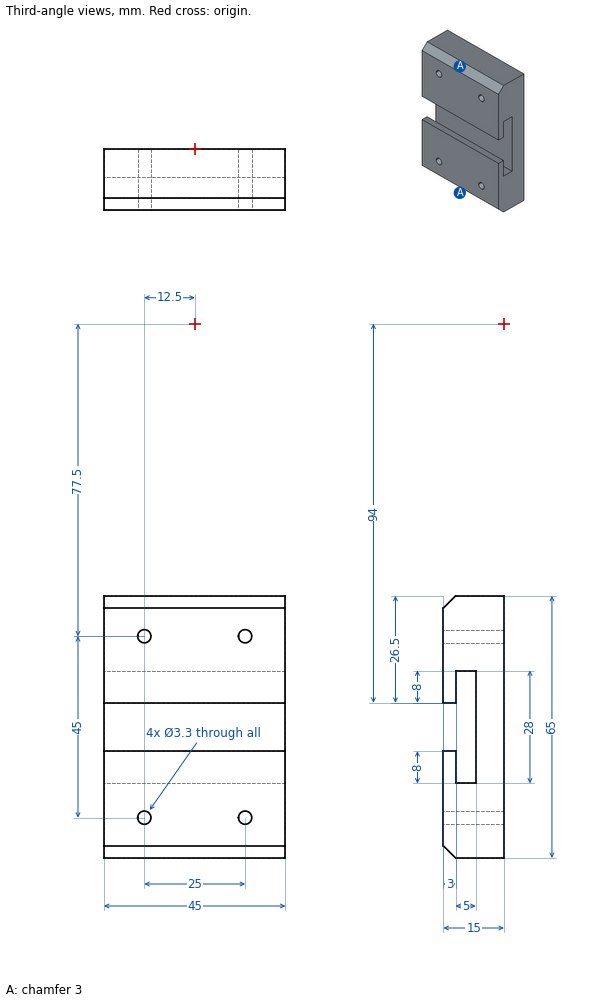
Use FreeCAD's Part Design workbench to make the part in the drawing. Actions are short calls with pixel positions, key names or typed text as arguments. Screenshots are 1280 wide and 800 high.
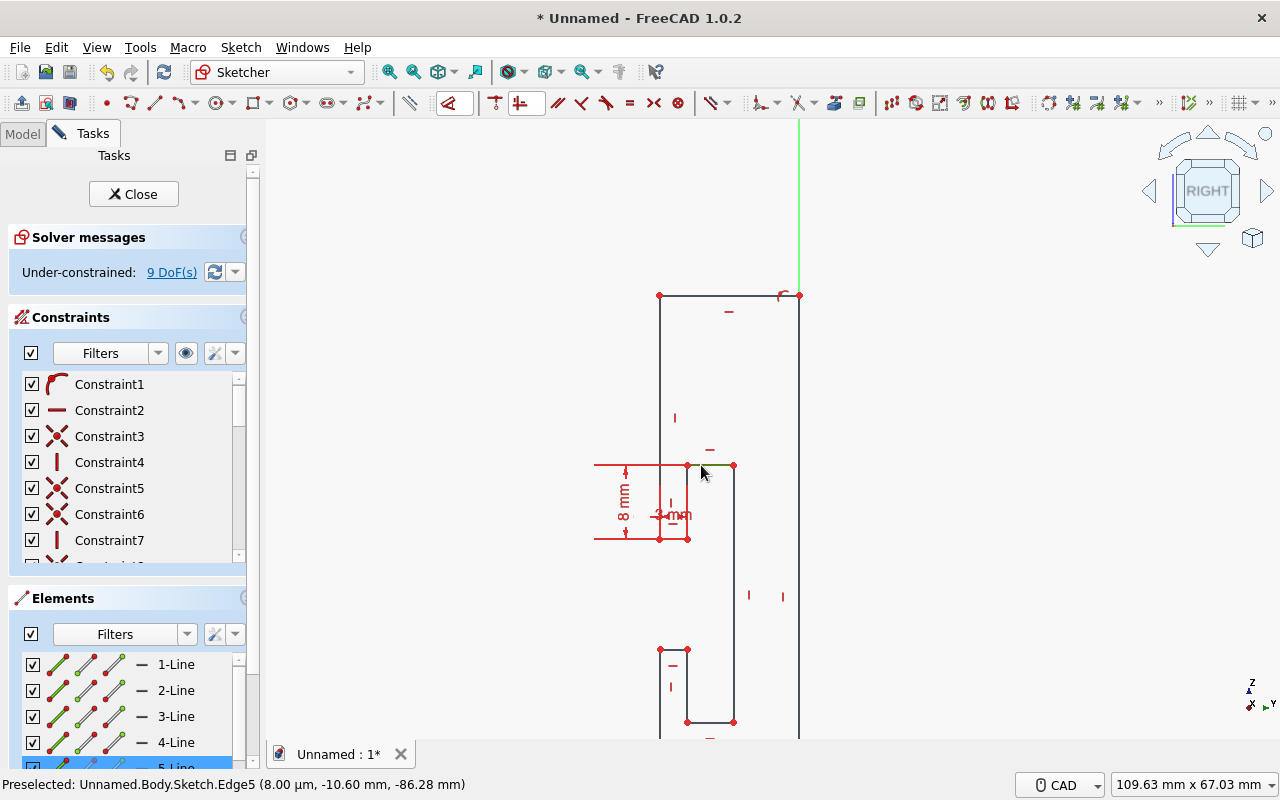
key(l)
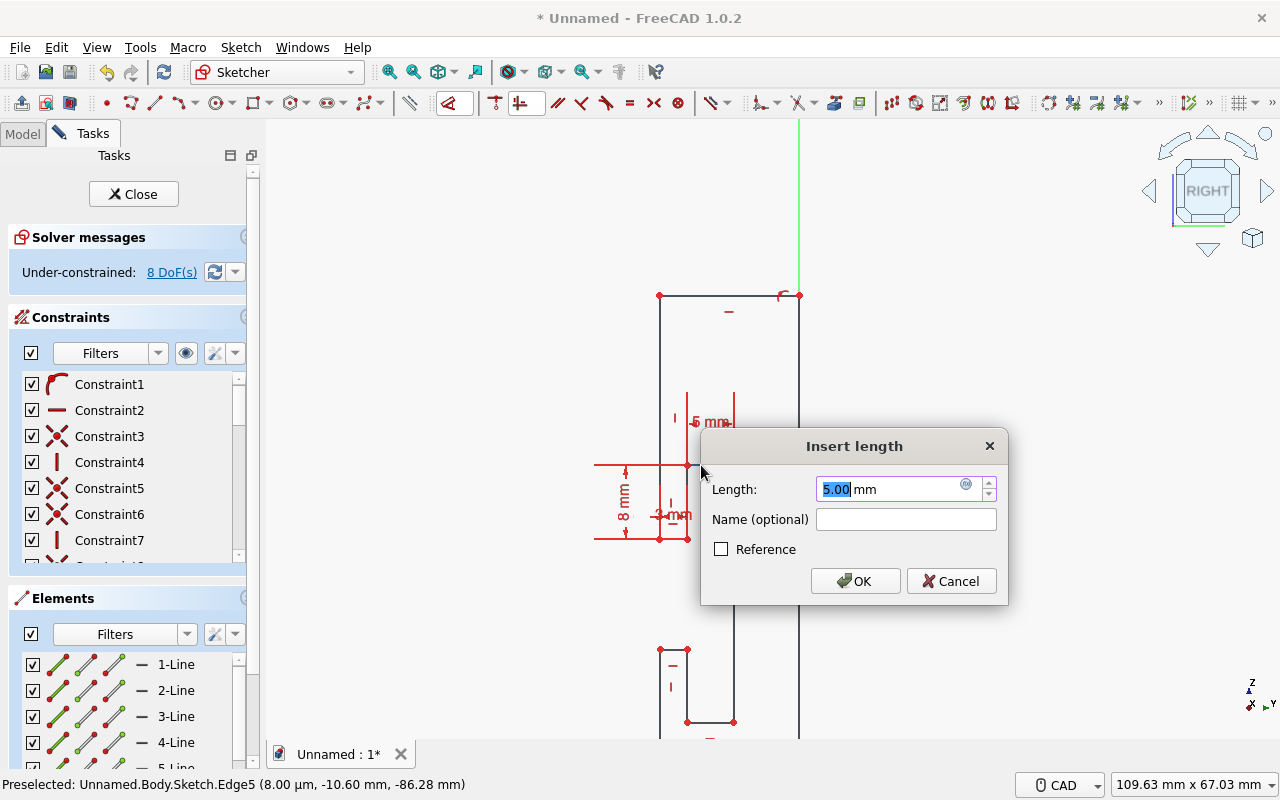
text(5)
key(Return)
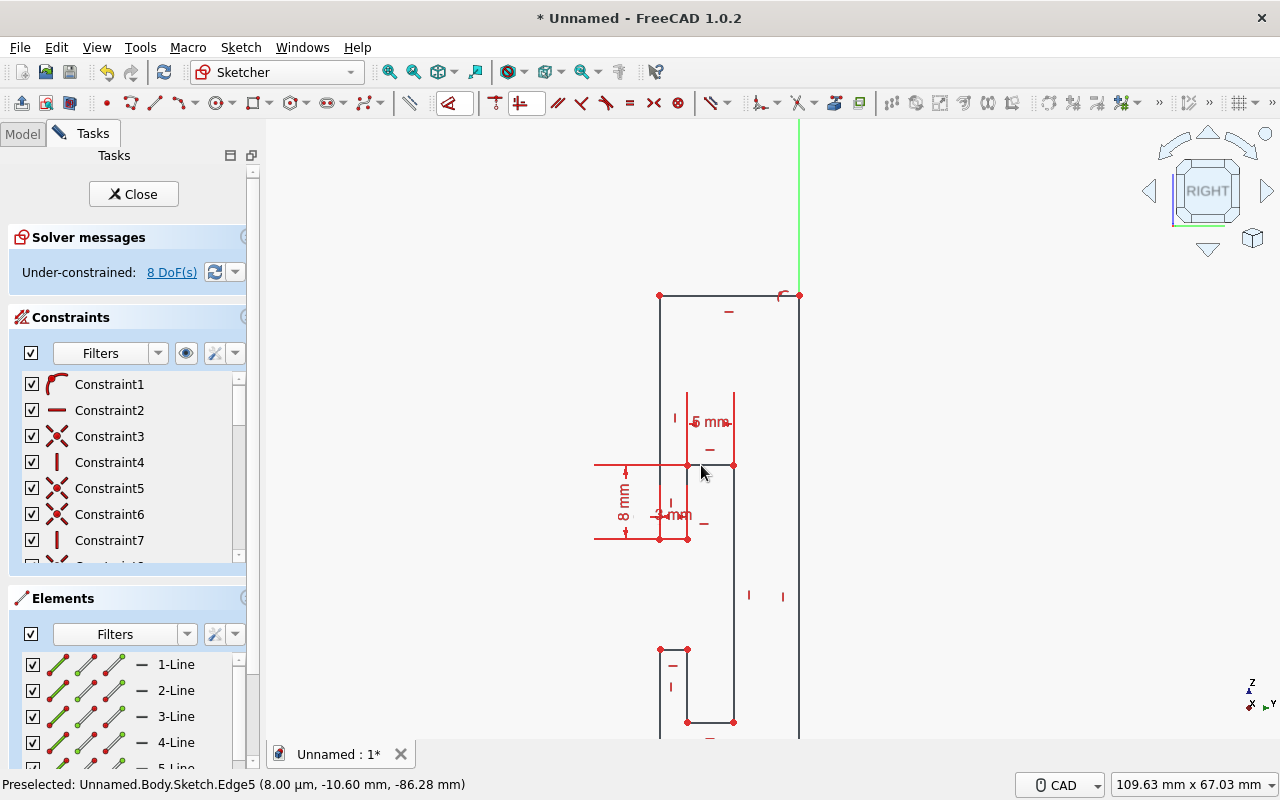
scroll(694, 493, down, 6)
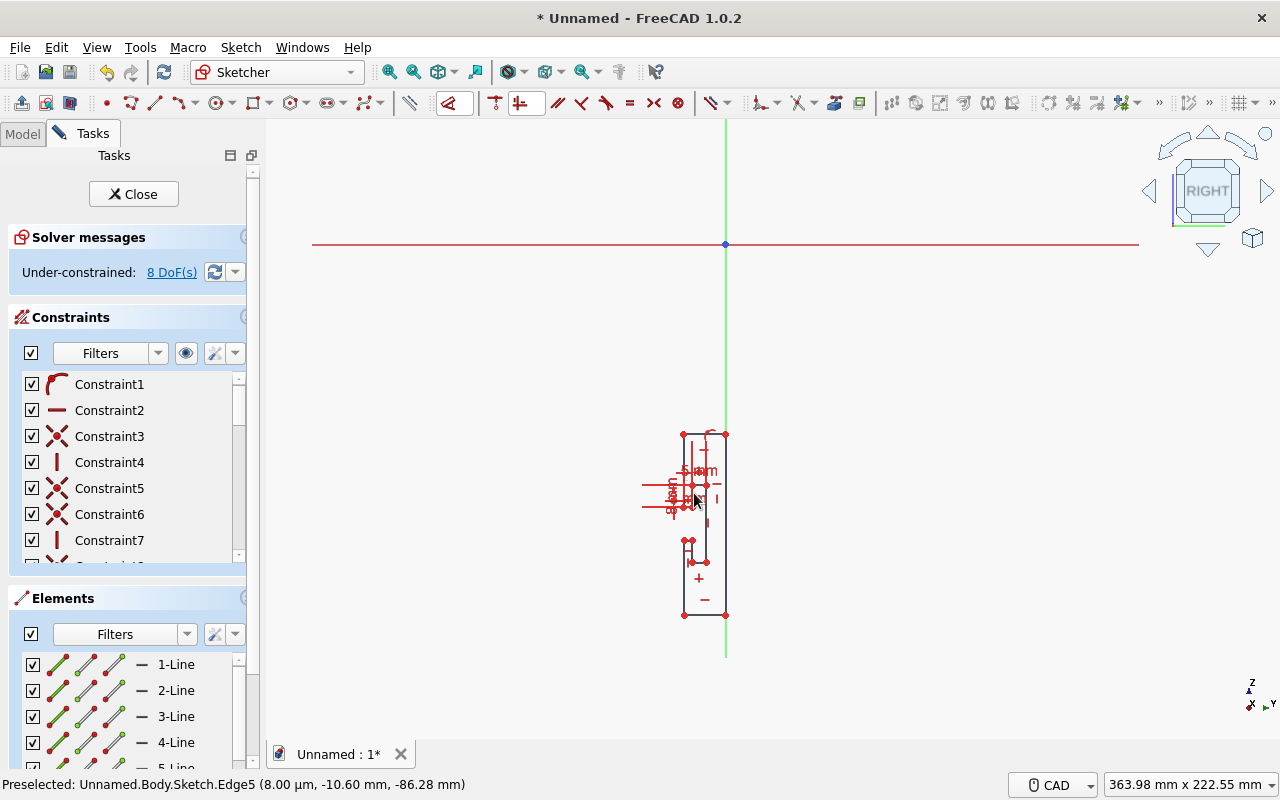
scroll(702, 563, up, 6)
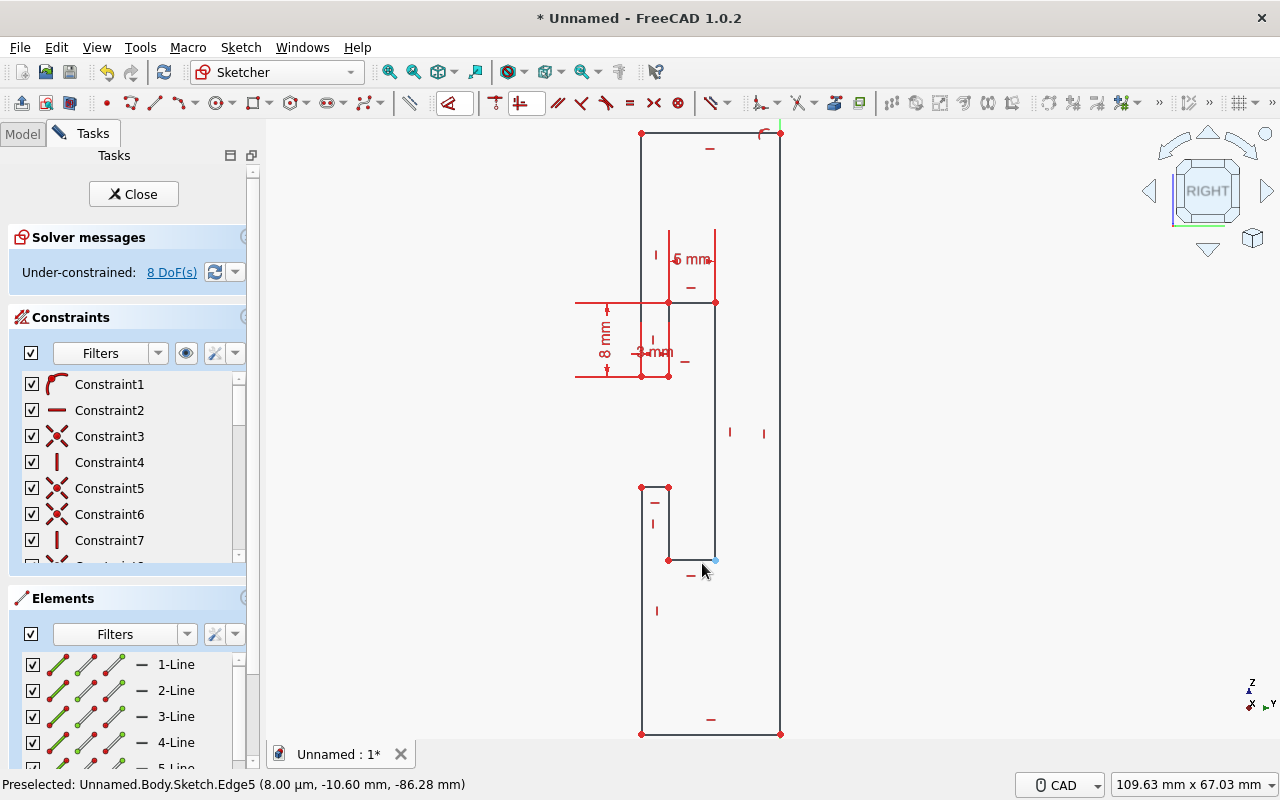
click(701, 560)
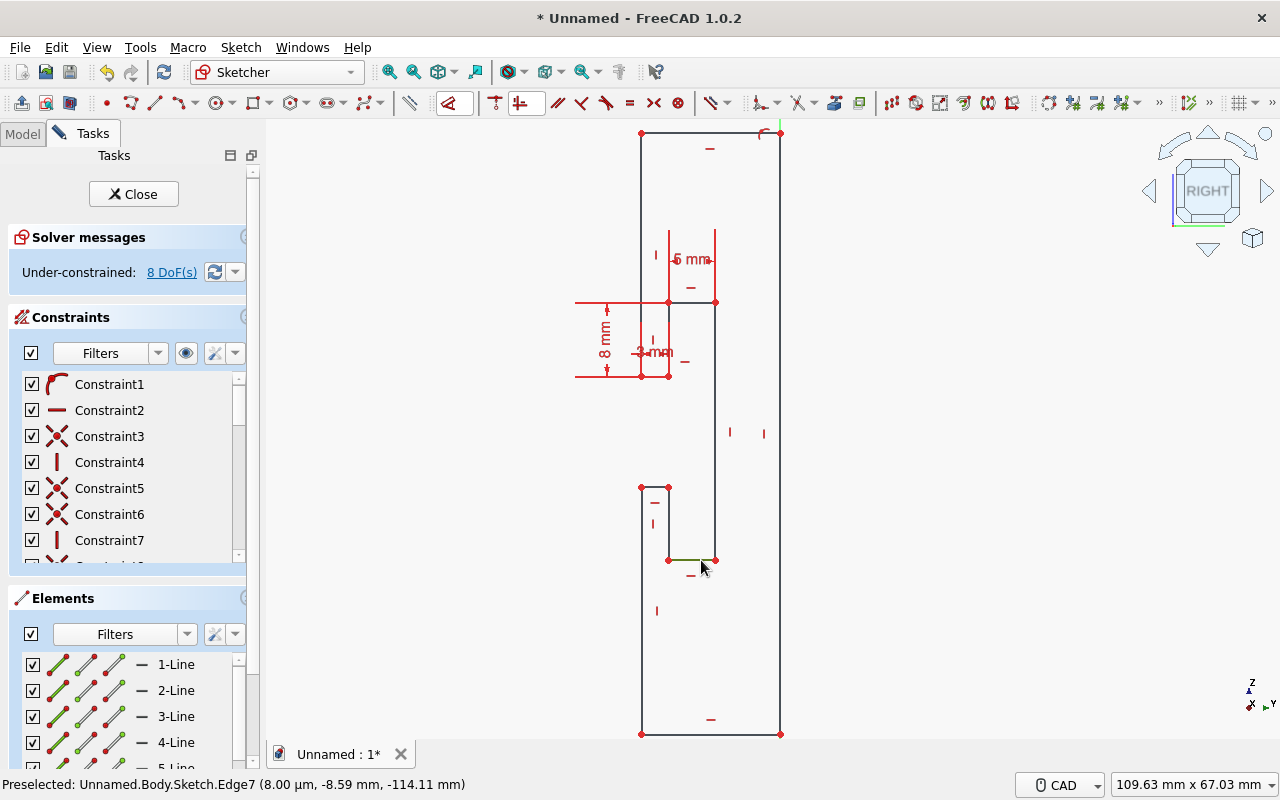
key(l)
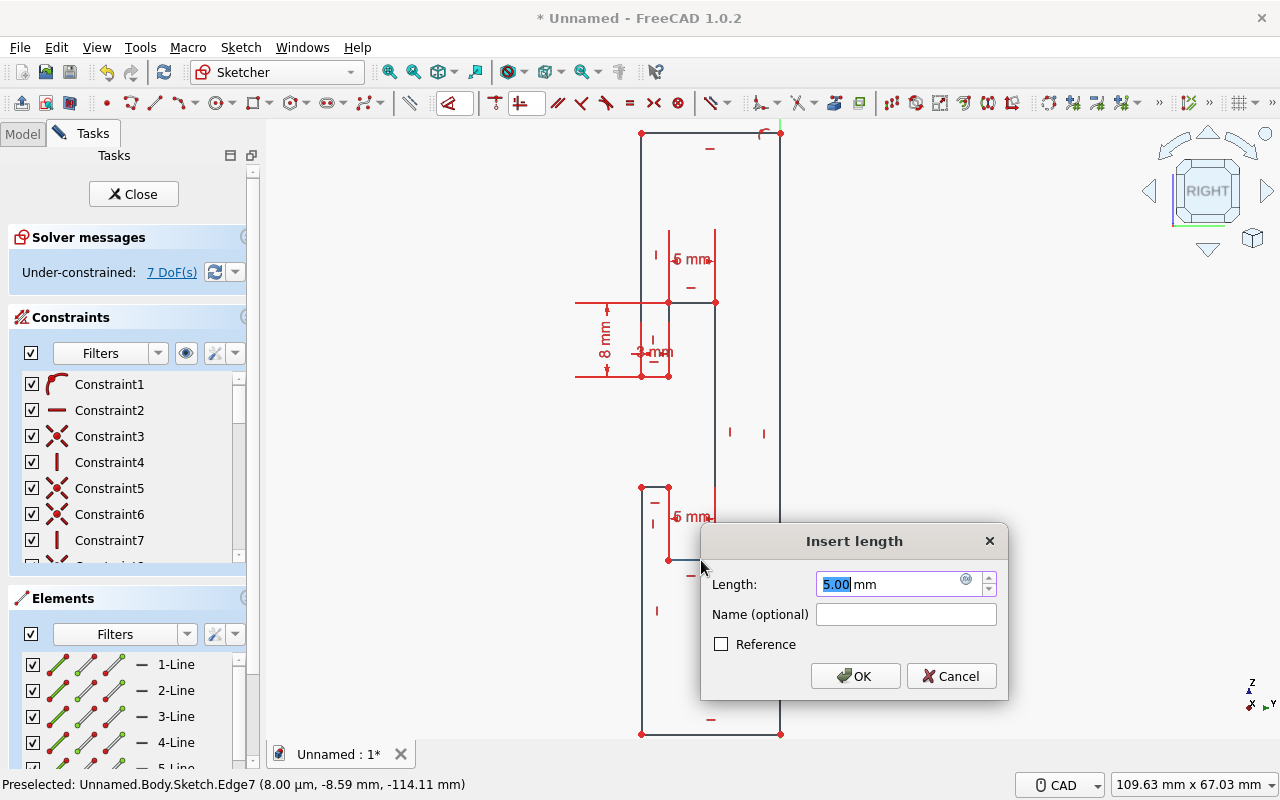
text(5)
key(Return)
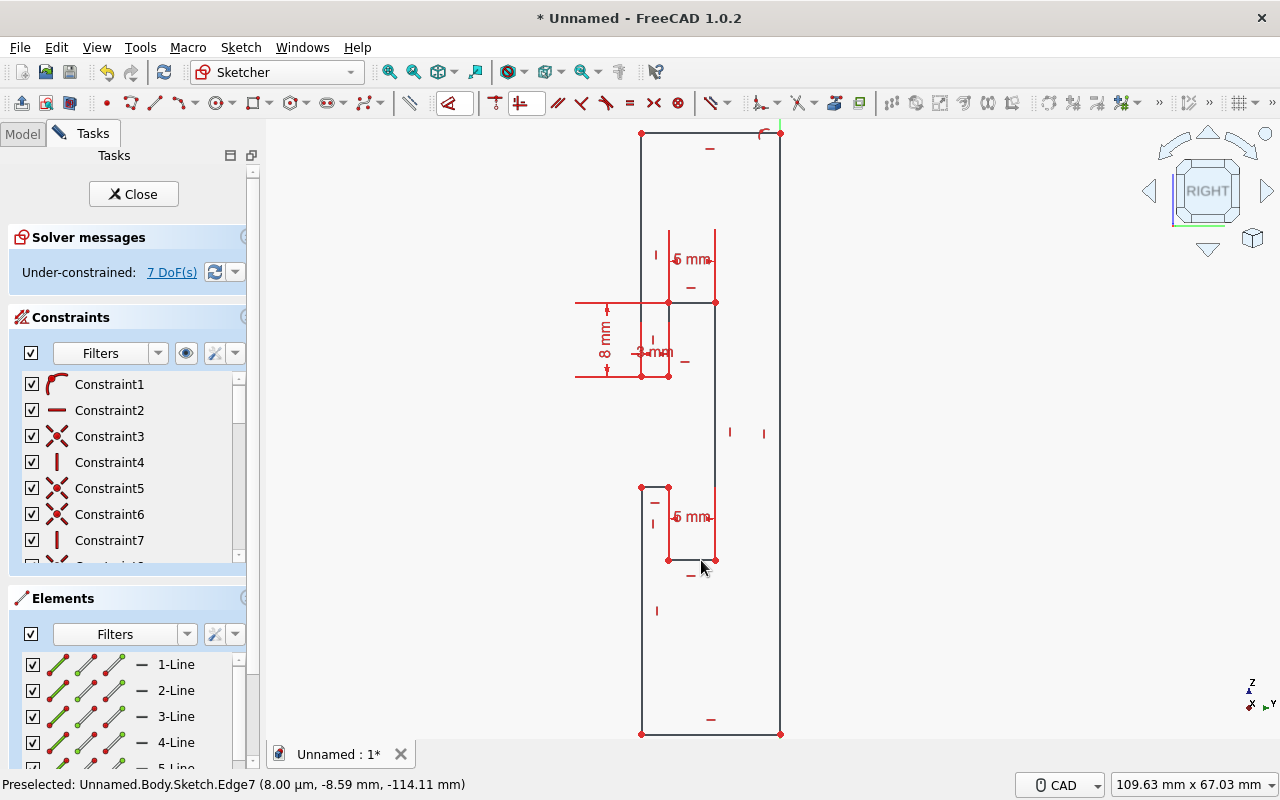
click(669, 538)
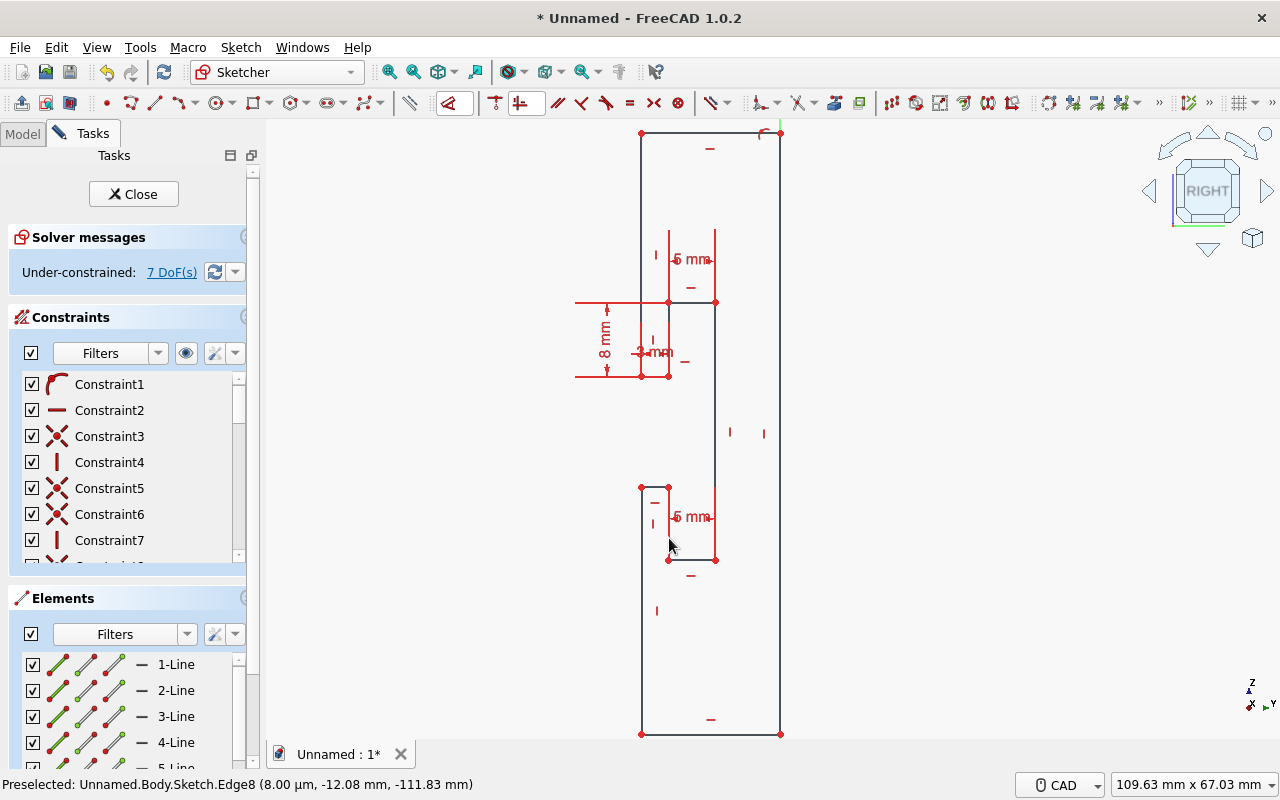
key(i)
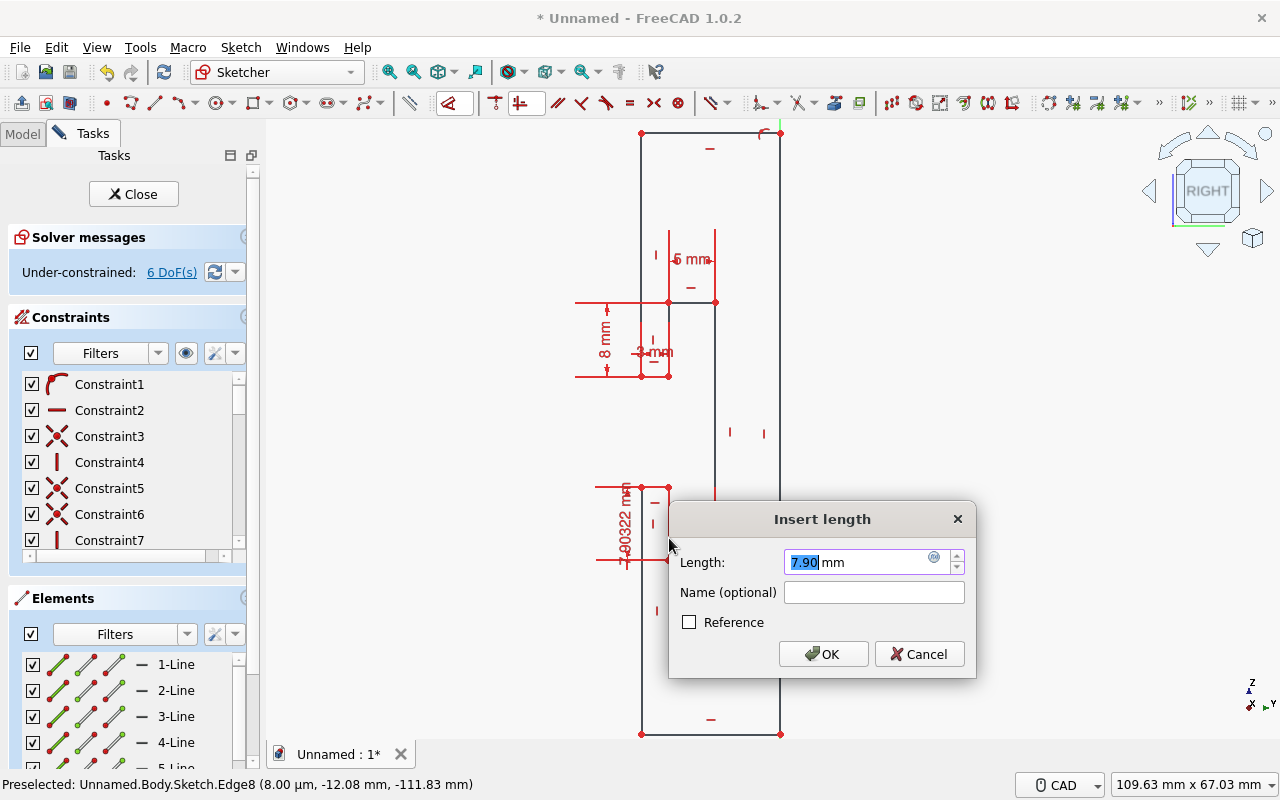
text(8)
key(Return)